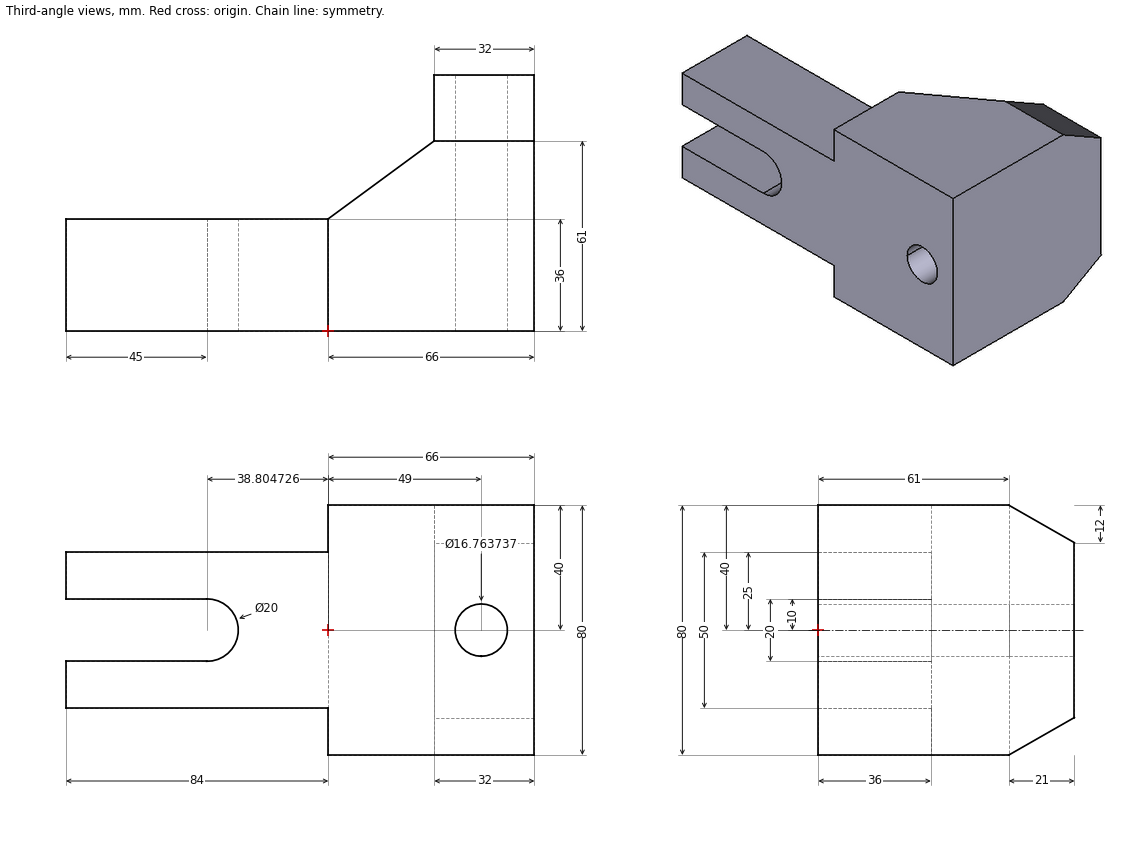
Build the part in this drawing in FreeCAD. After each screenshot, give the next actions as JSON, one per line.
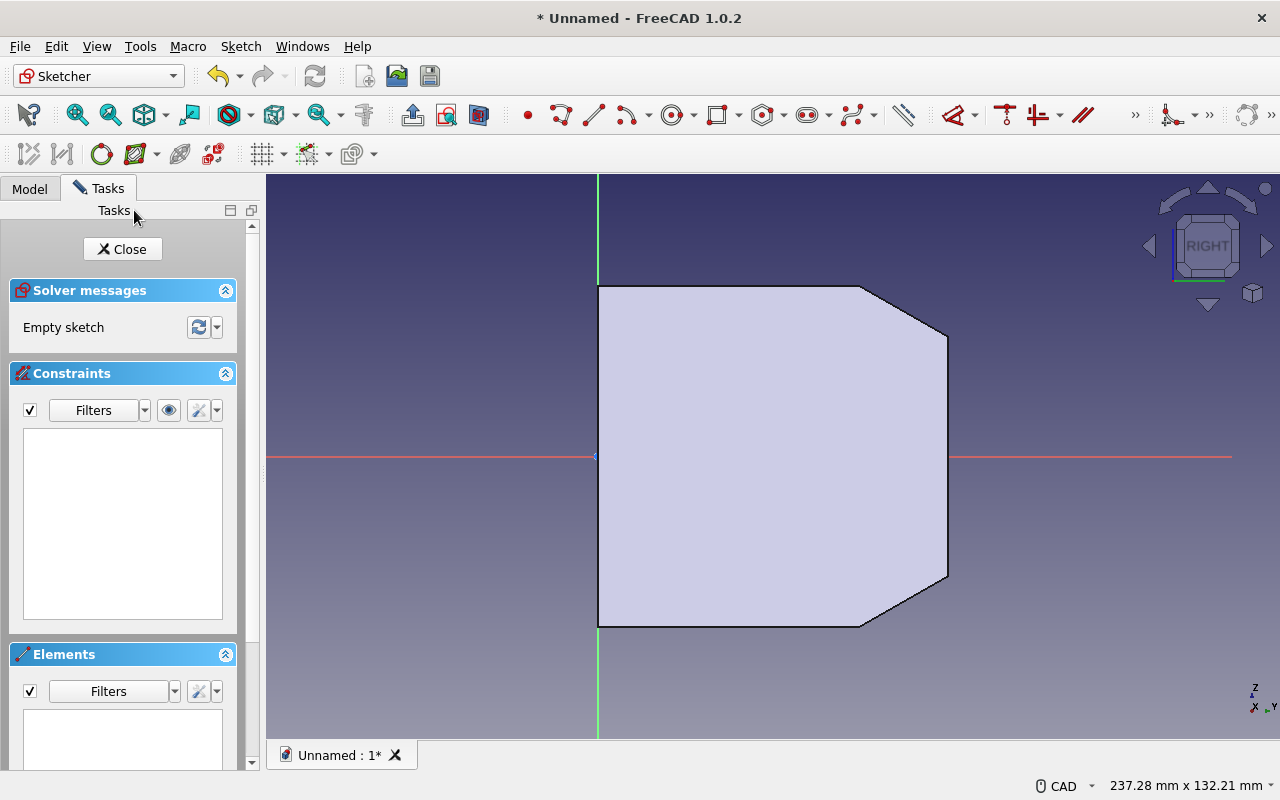
{"action": "key", "text": "q s"}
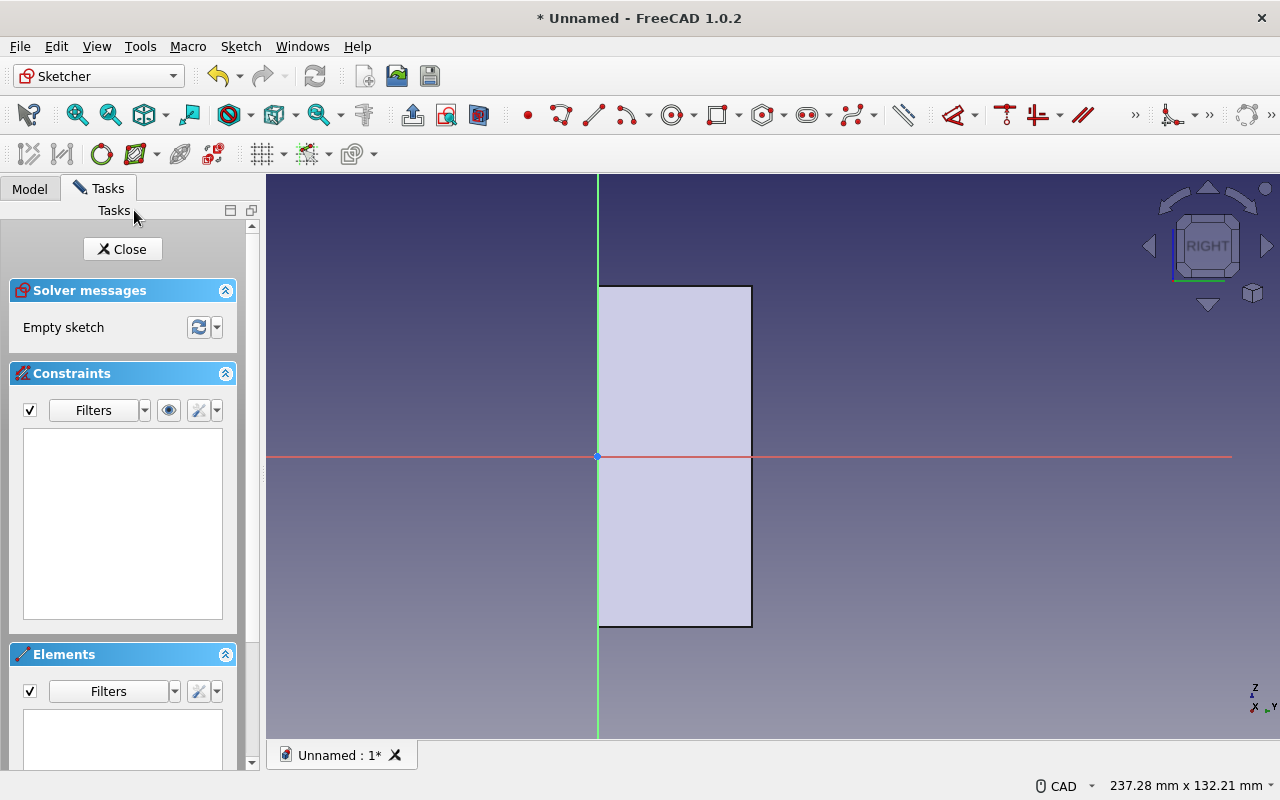
{"action": "scroll", "coordinate": [638, 456], "scroll_direction": "up", "scroll_amount": 3}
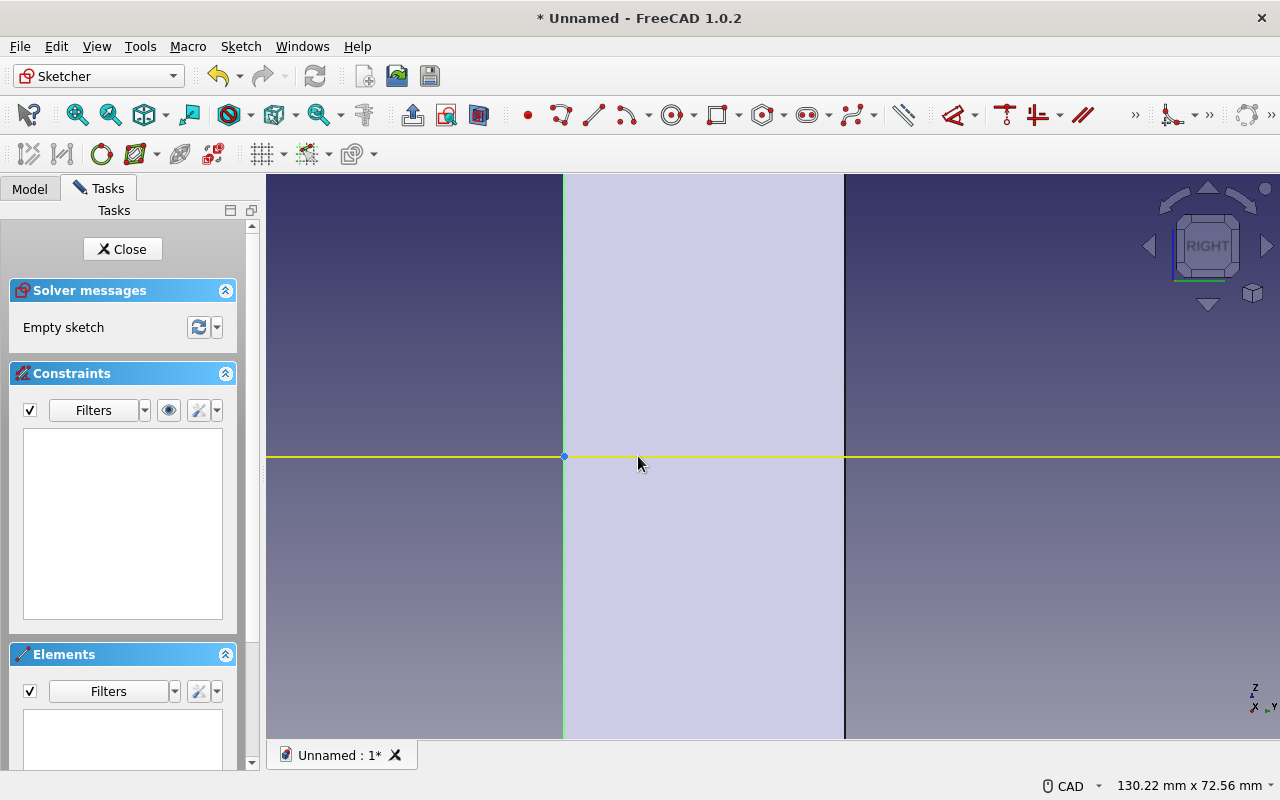
{"action": "key", "text": "g r"}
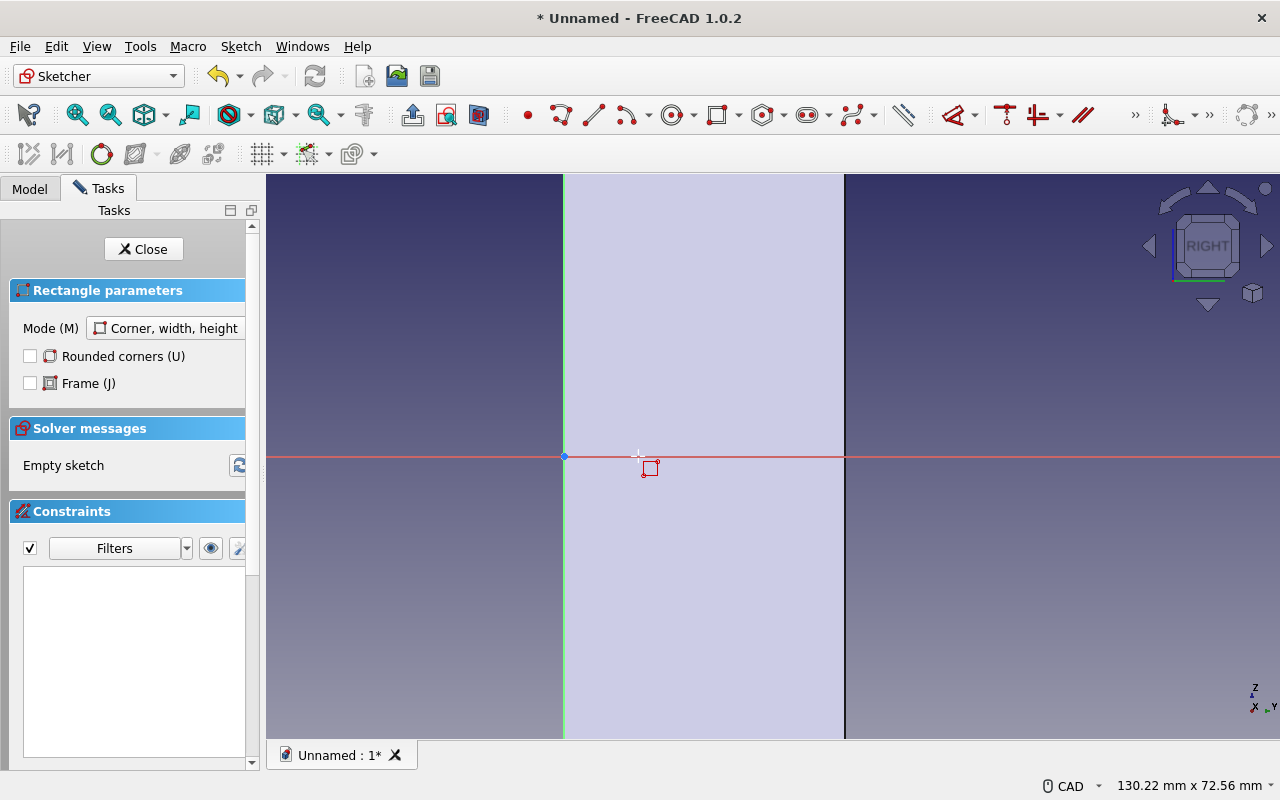
{"action": "left_click", "coordinate": [564, 262]}
{"action": "left_click", "coordinate": [845, 651]}
{"action": "key", "text": "Escape"}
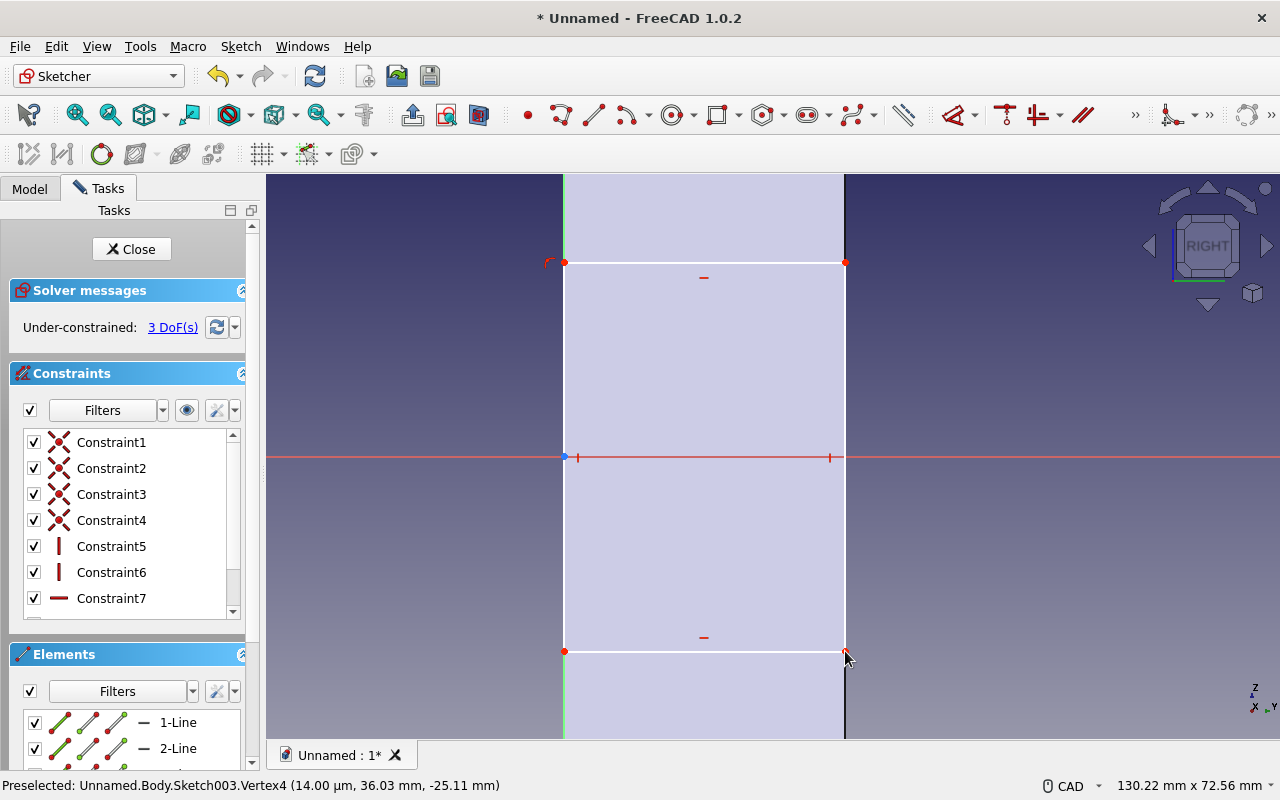
{"action": "key", "text": "d"}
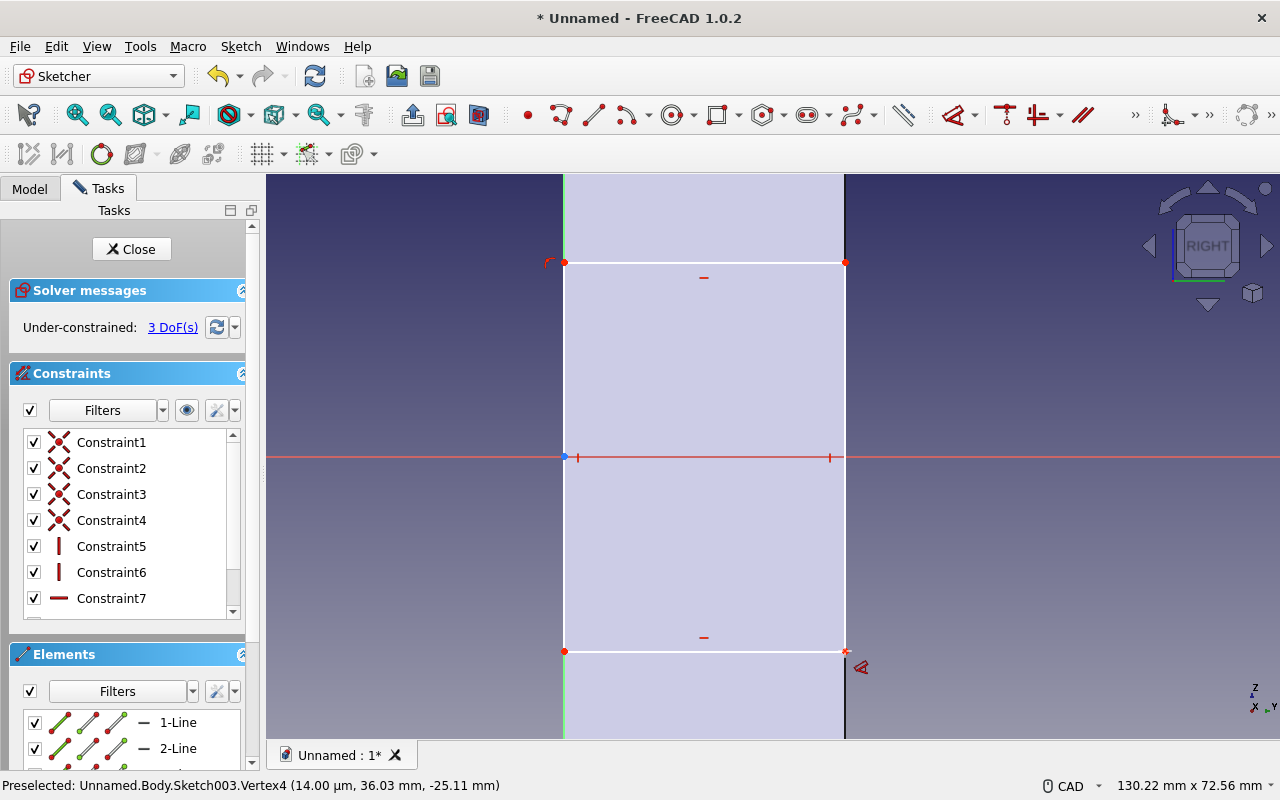
{"action": "left_click", "coordinate": [564, 380]}
{"action": "left_click", "coordinate": [530, 368]}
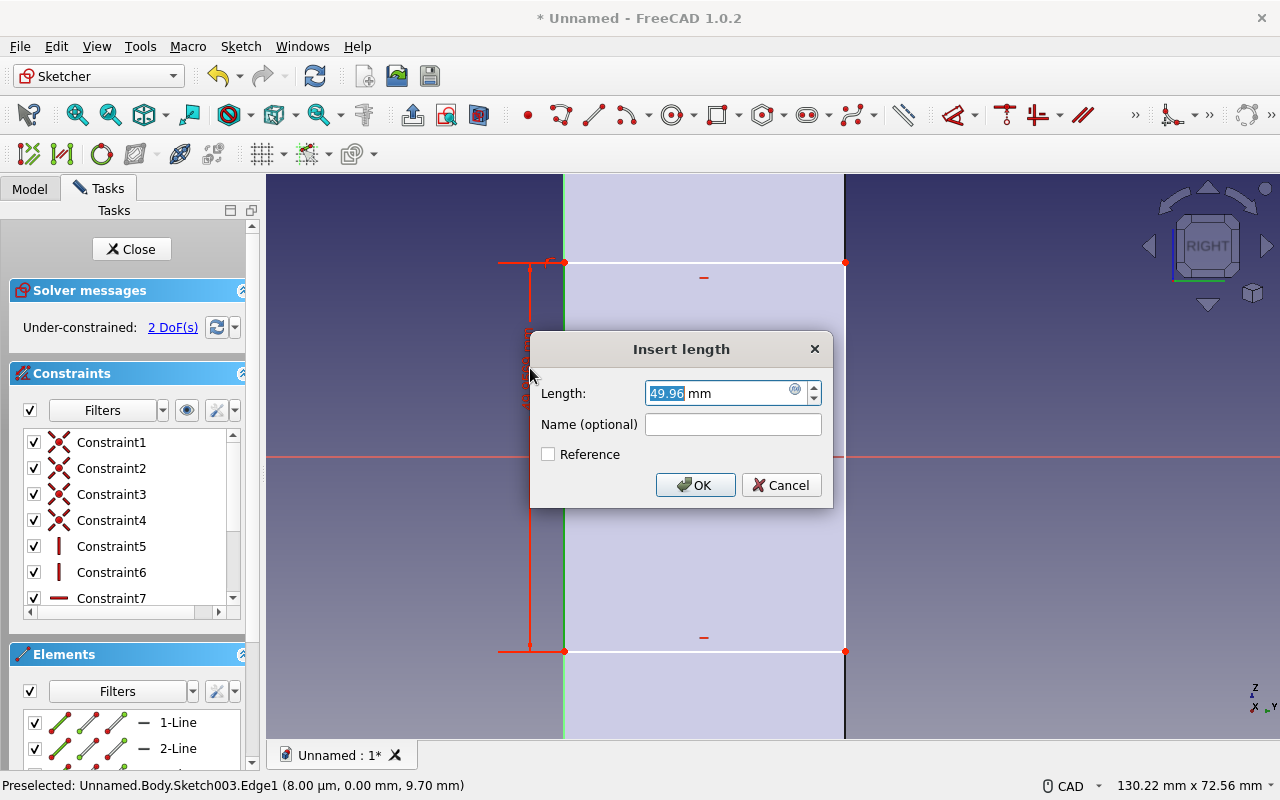
{"action": "type", "text": "50"}
{"action": "key", "text": "Return"}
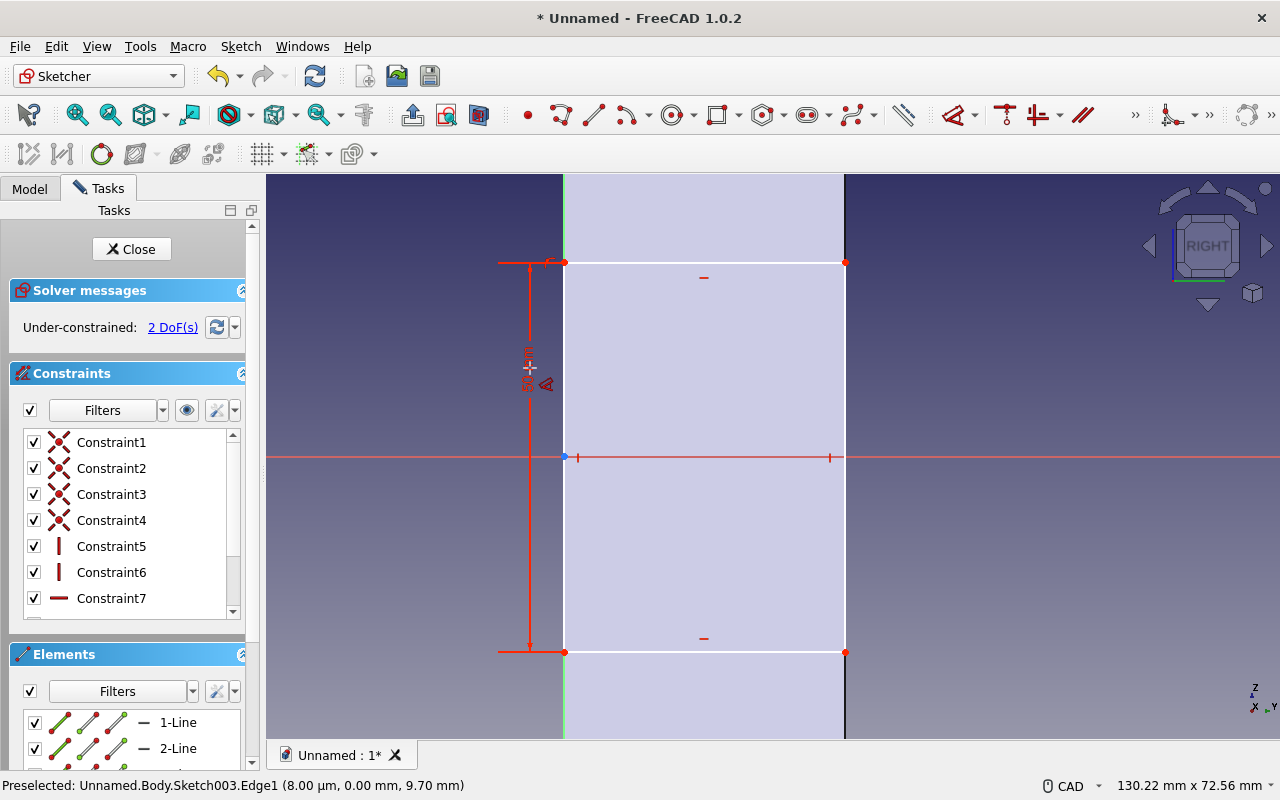
{"action": "left_click", "coordinate": [649, 652]}
{"action": "left_click", "coordinate": [705, 686]}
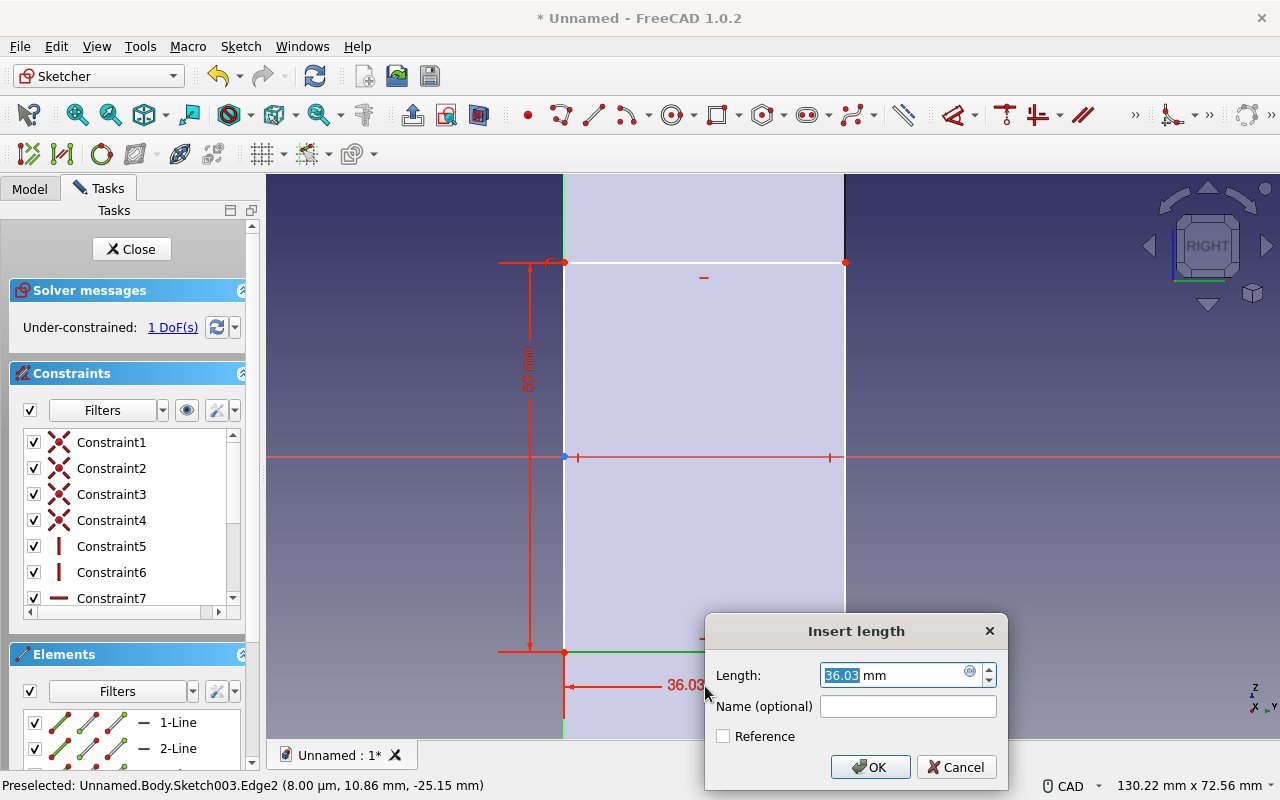
{"action": "type", "text": "36"}
{"action": "key", "text": "Return"}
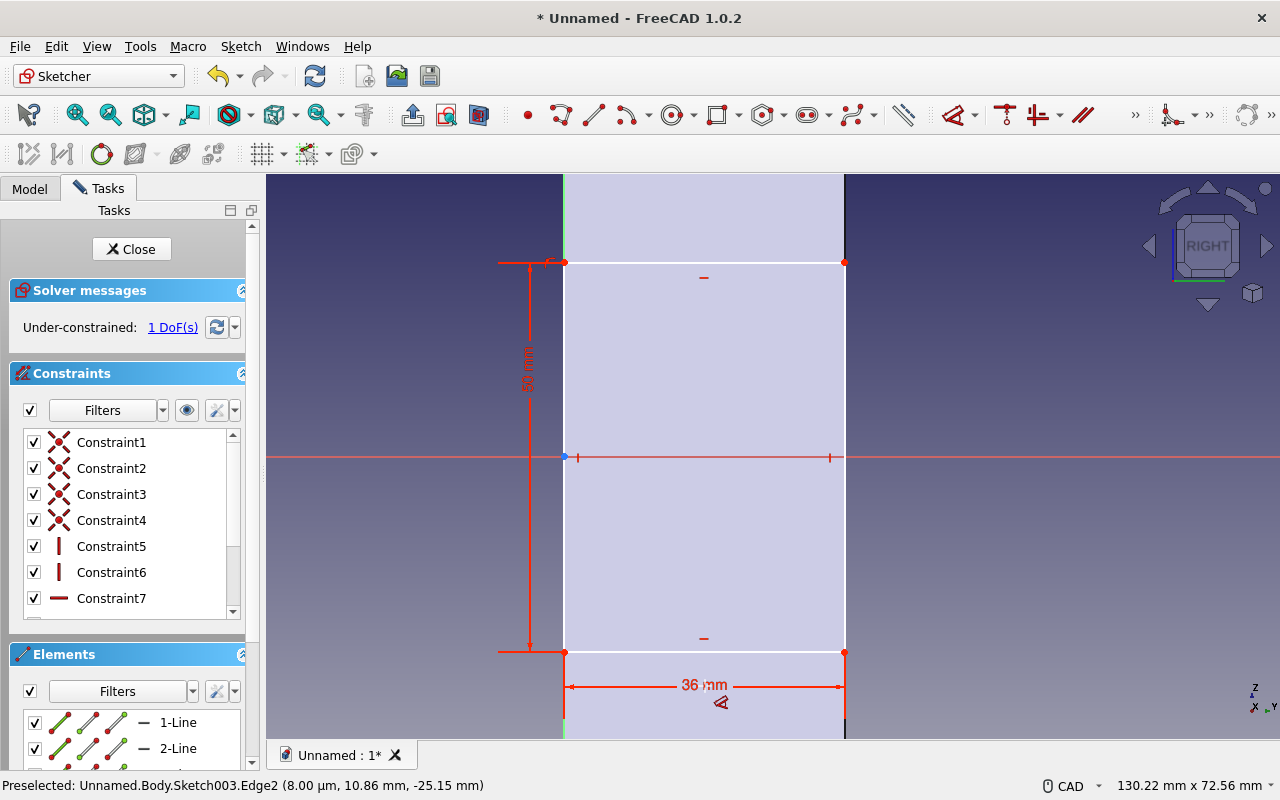
{"action": "left_click", "coordinate": [564, 263]}
{"action": "left_click", "coordinate": [530, 315]}